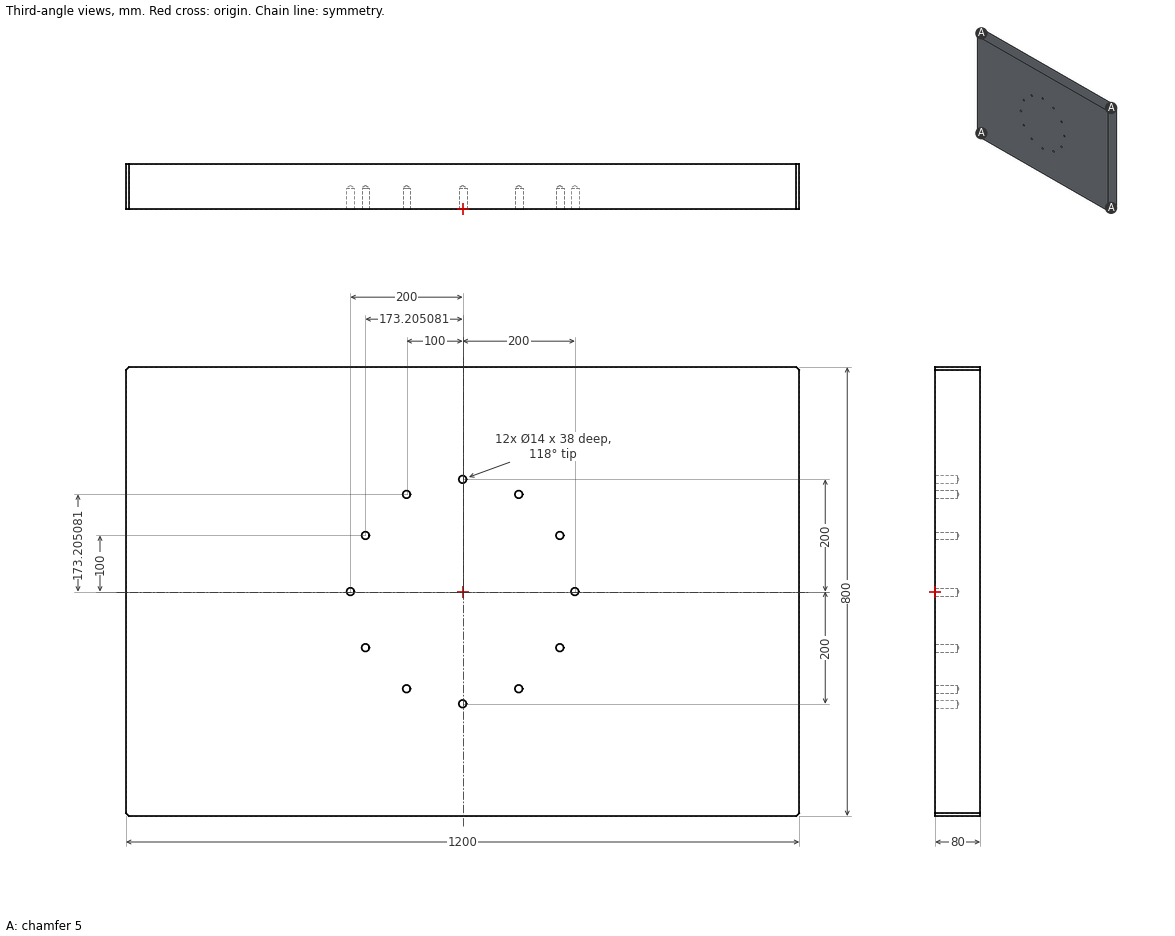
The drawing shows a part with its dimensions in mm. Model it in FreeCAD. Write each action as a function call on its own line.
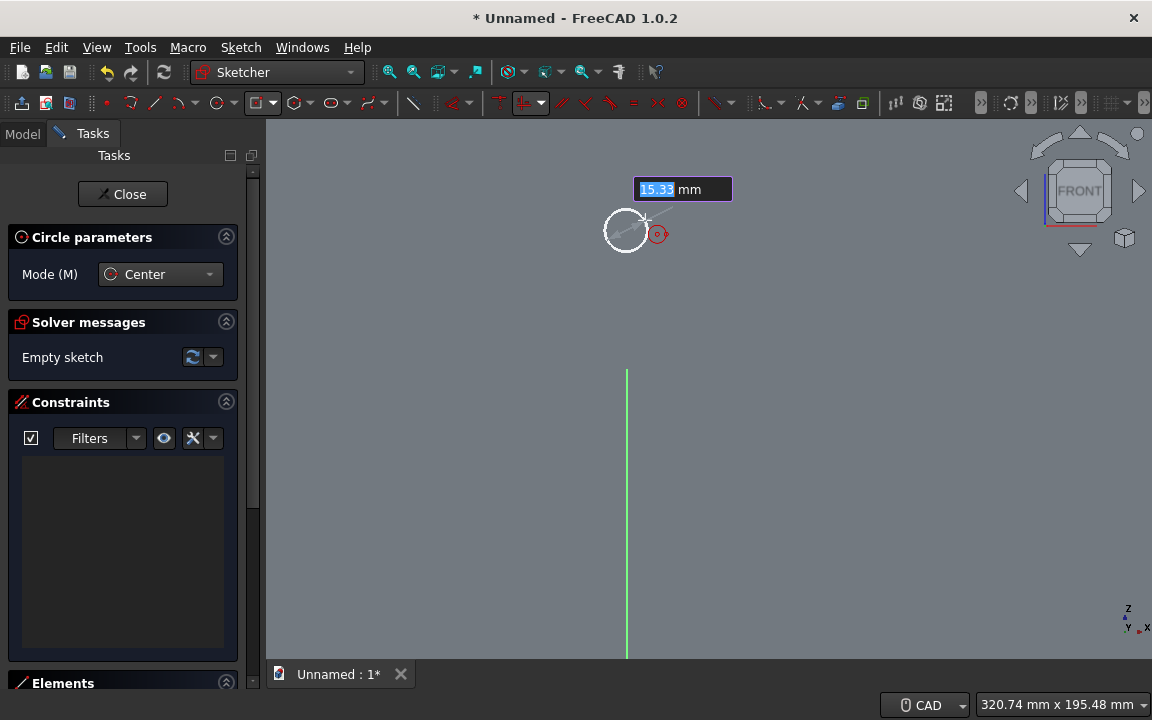
text(14)
key(Return)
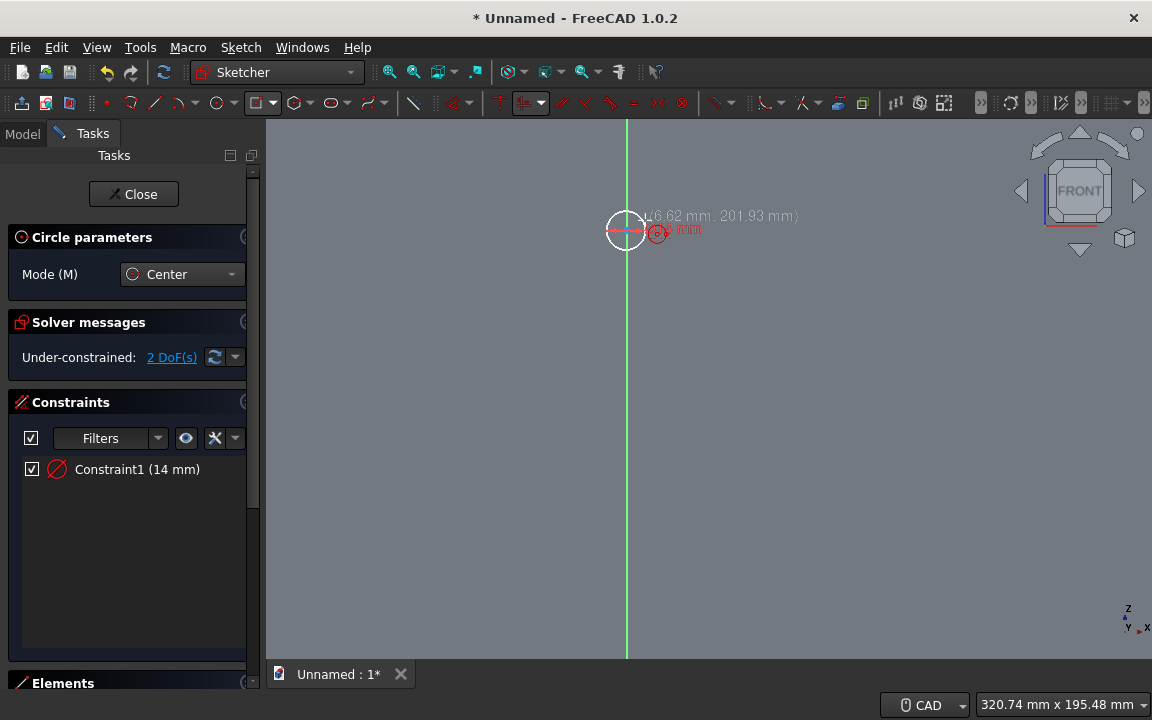
click(350, 300)
move(364, 287)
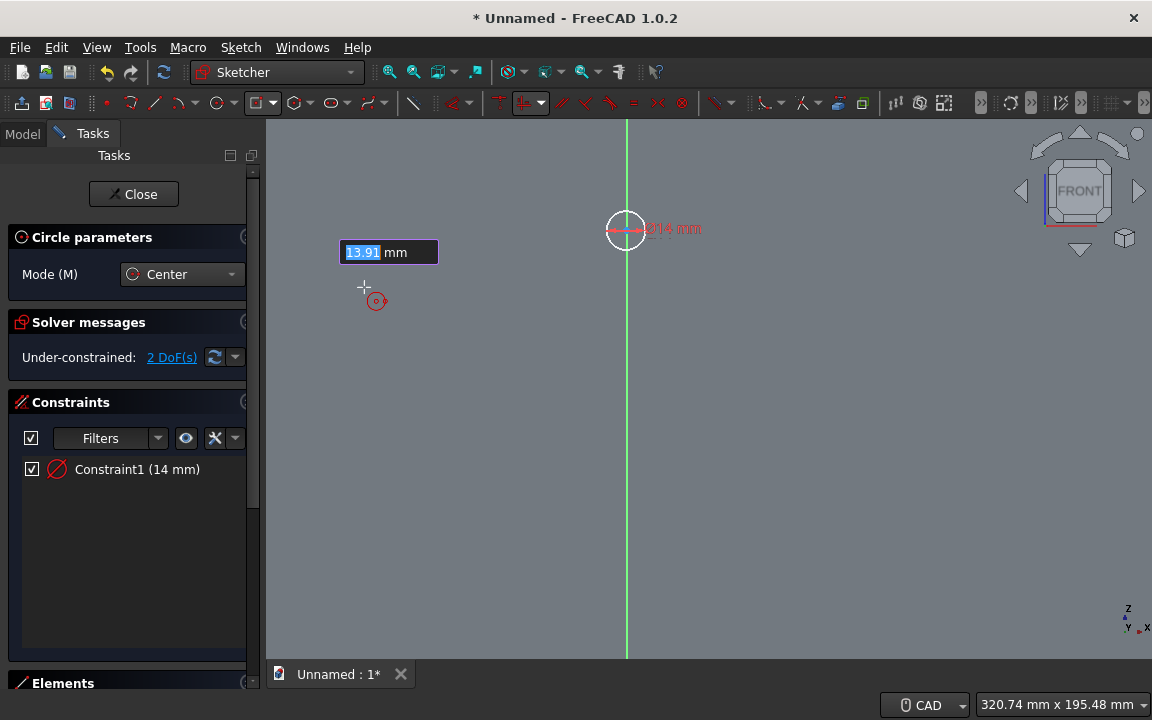
text(14)
key(Return)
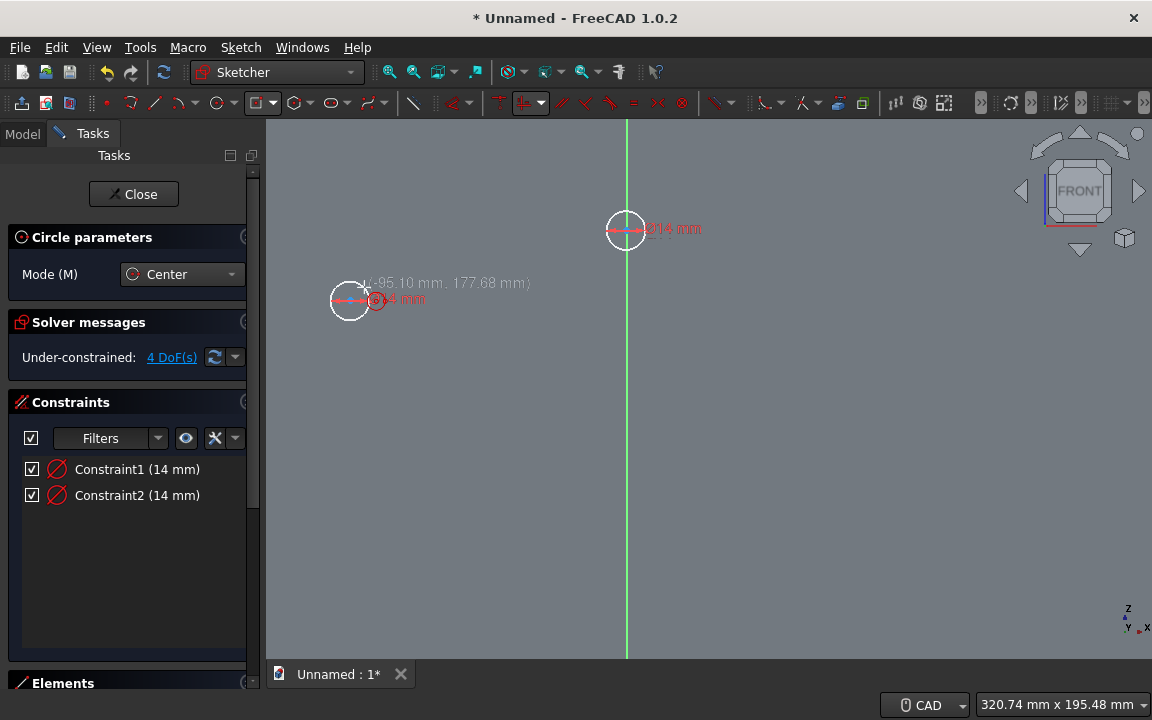
scroll(646, 221, down, 6)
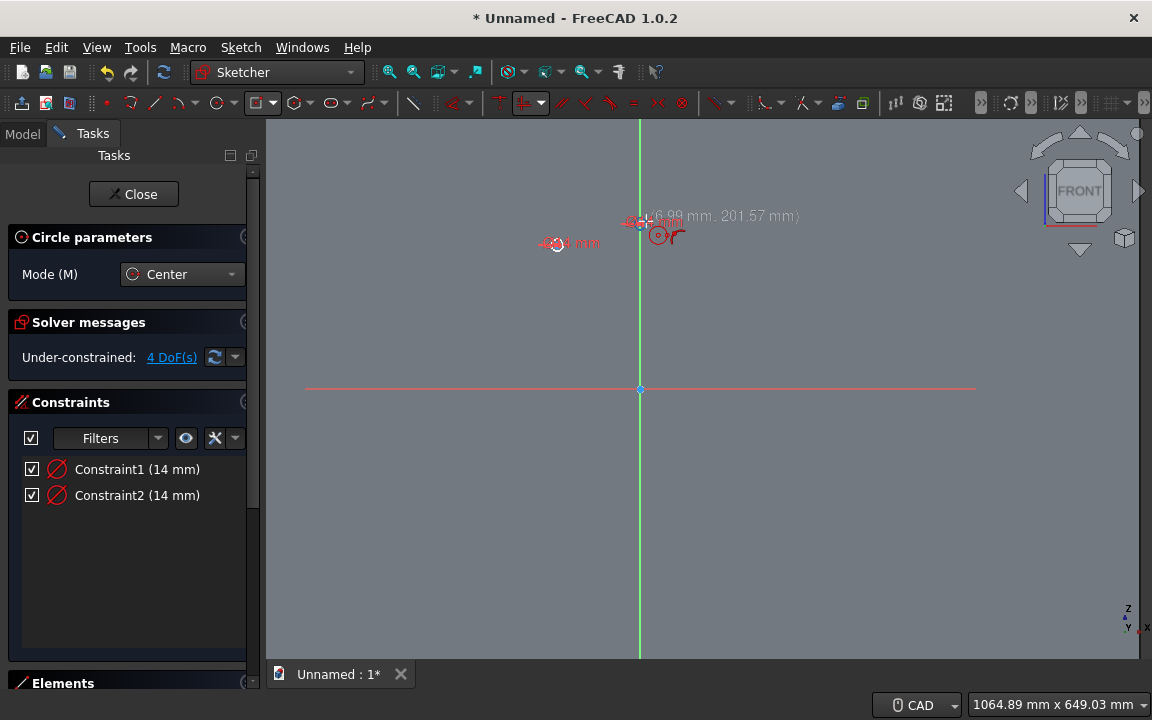
scroll(496, 306, up, 7)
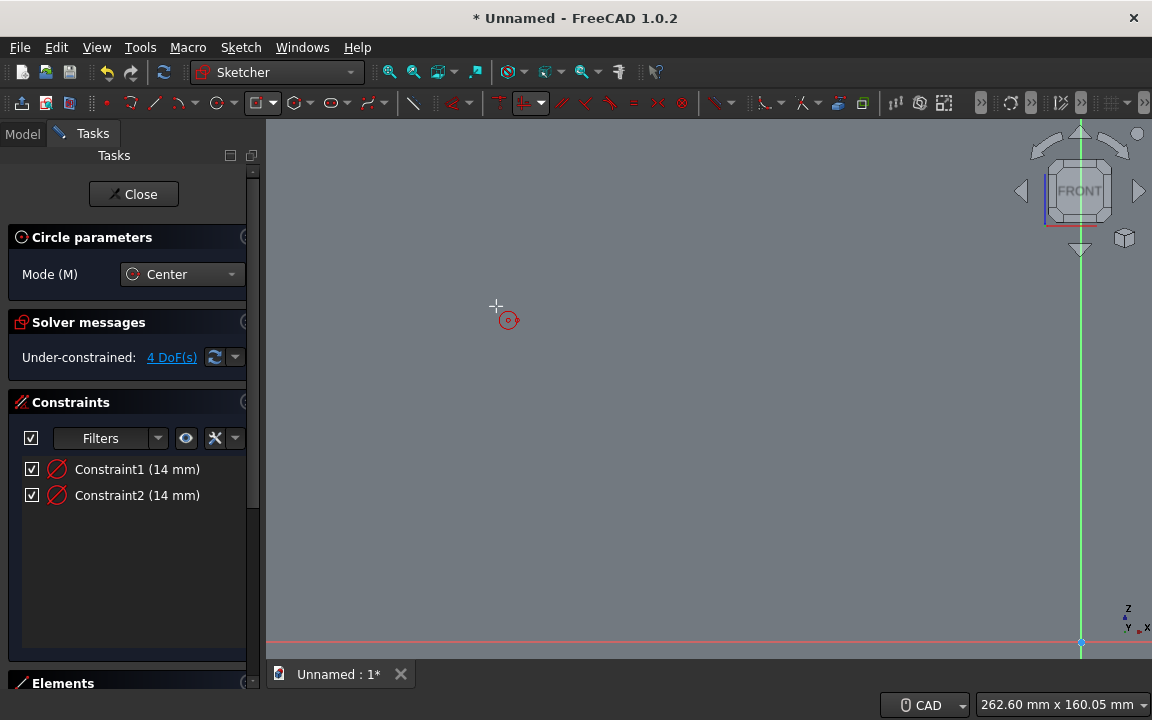
scroll(496, 306, down, 7)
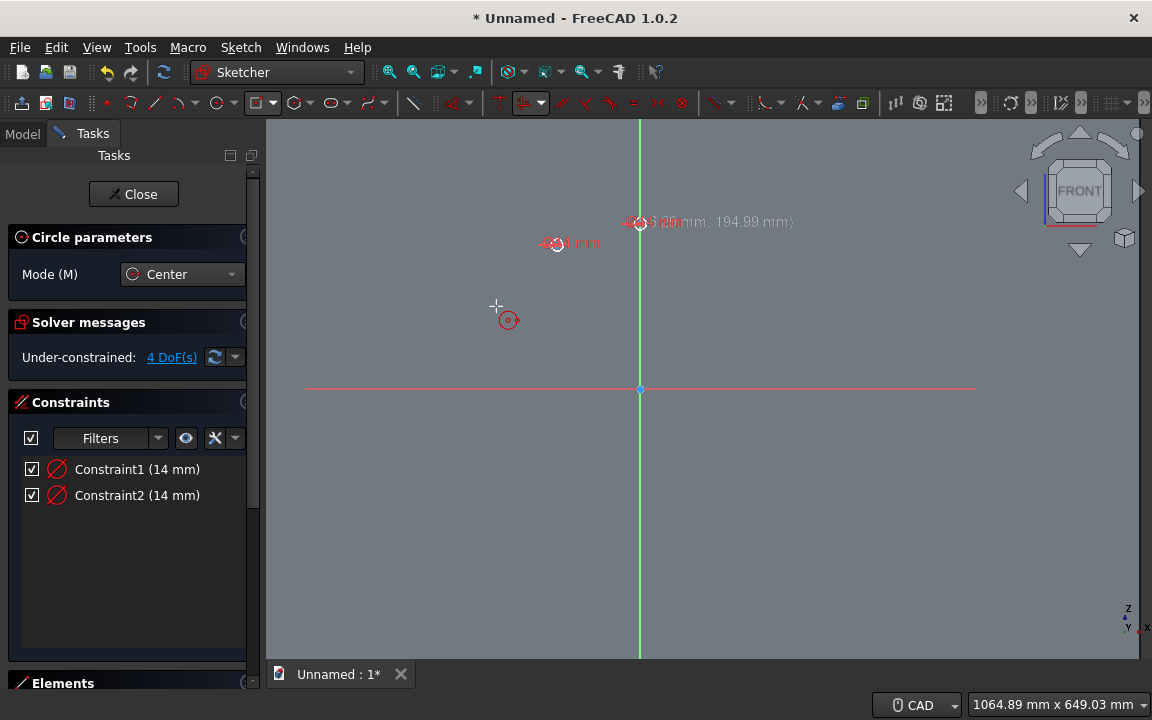
click(496, 306)
move(500, 302)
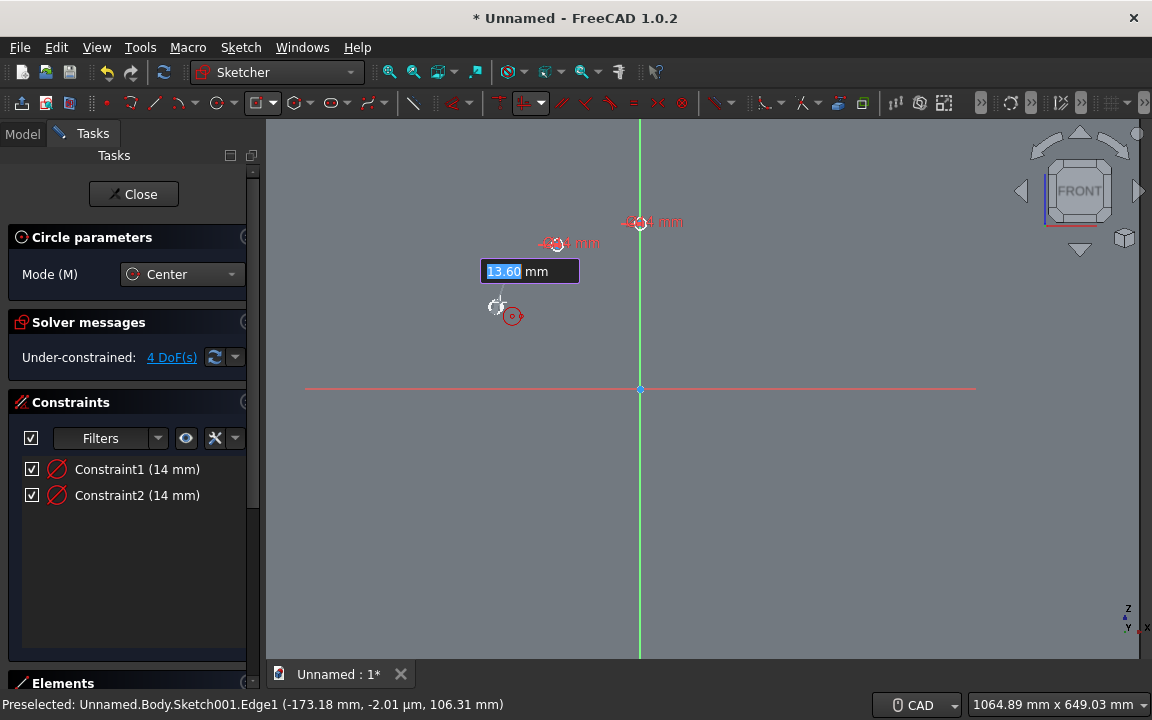
text(14)
key(Return)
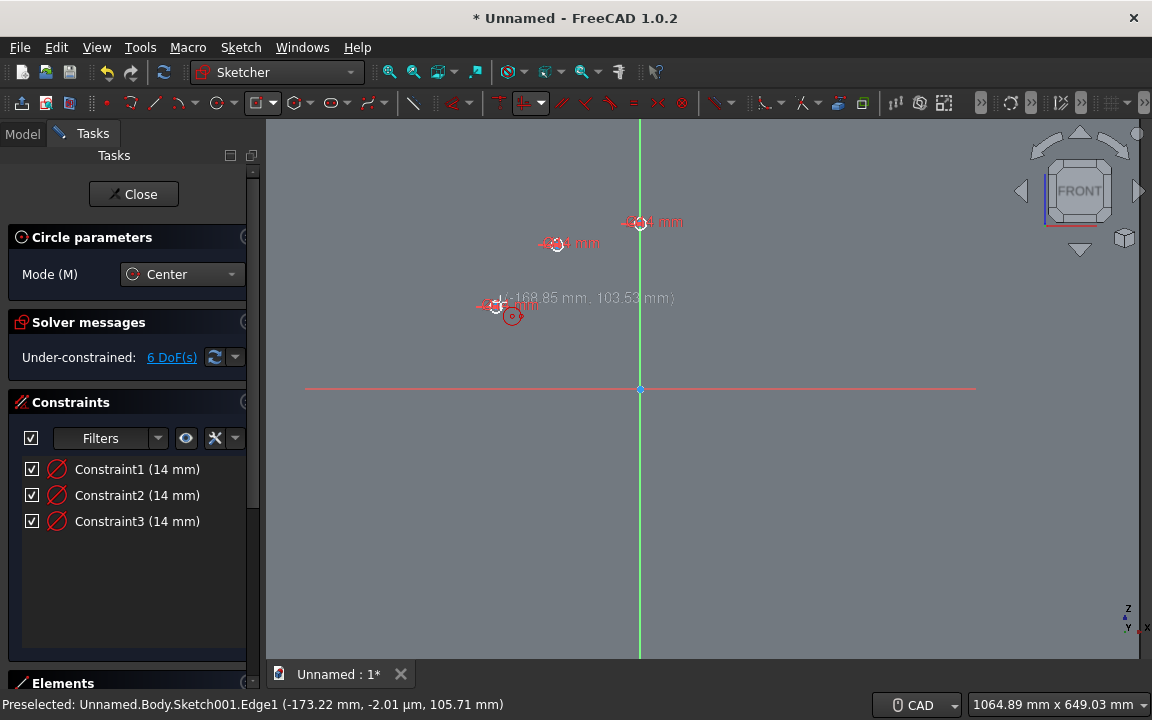
scroll(474, 389, up, 7)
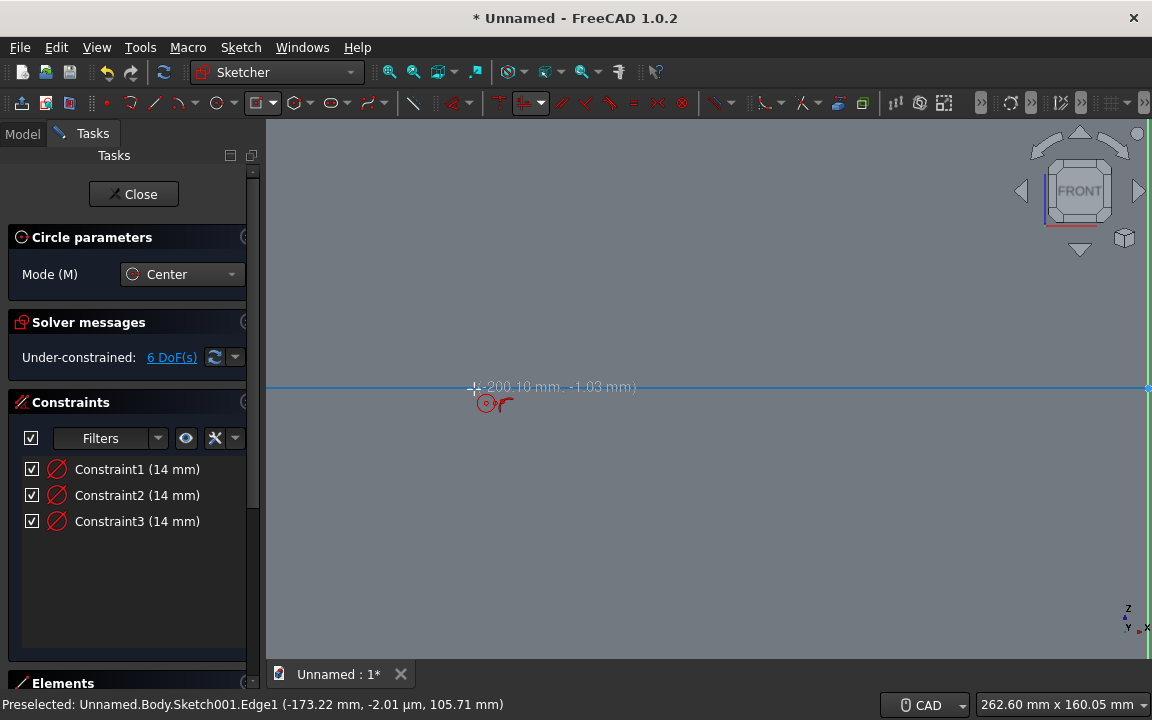
scroll(474, 389, down, 7)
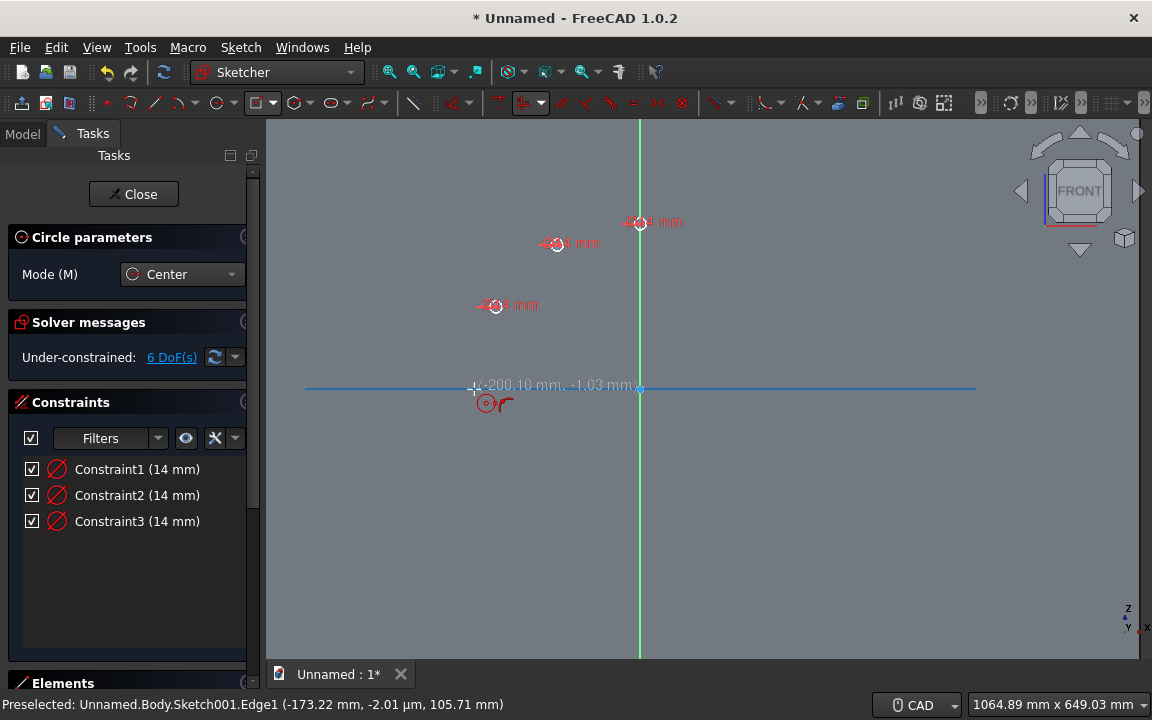
click(474, 389)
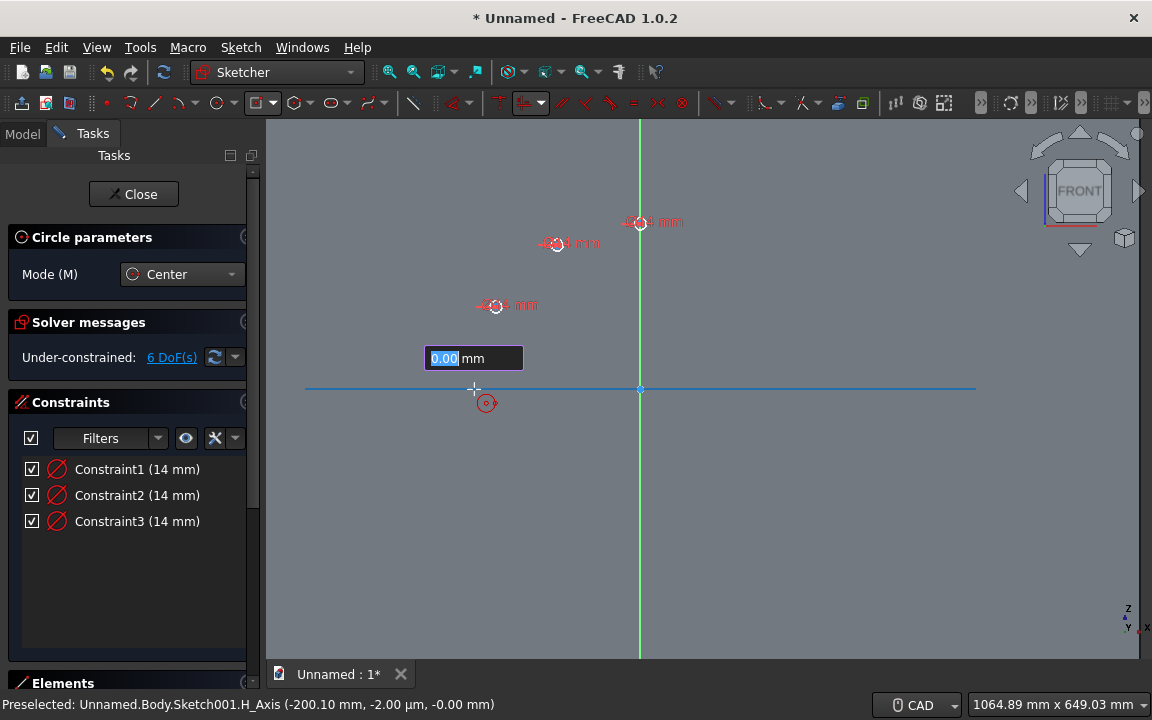
scroll(476, 384, up, 6)
move(476, 382)